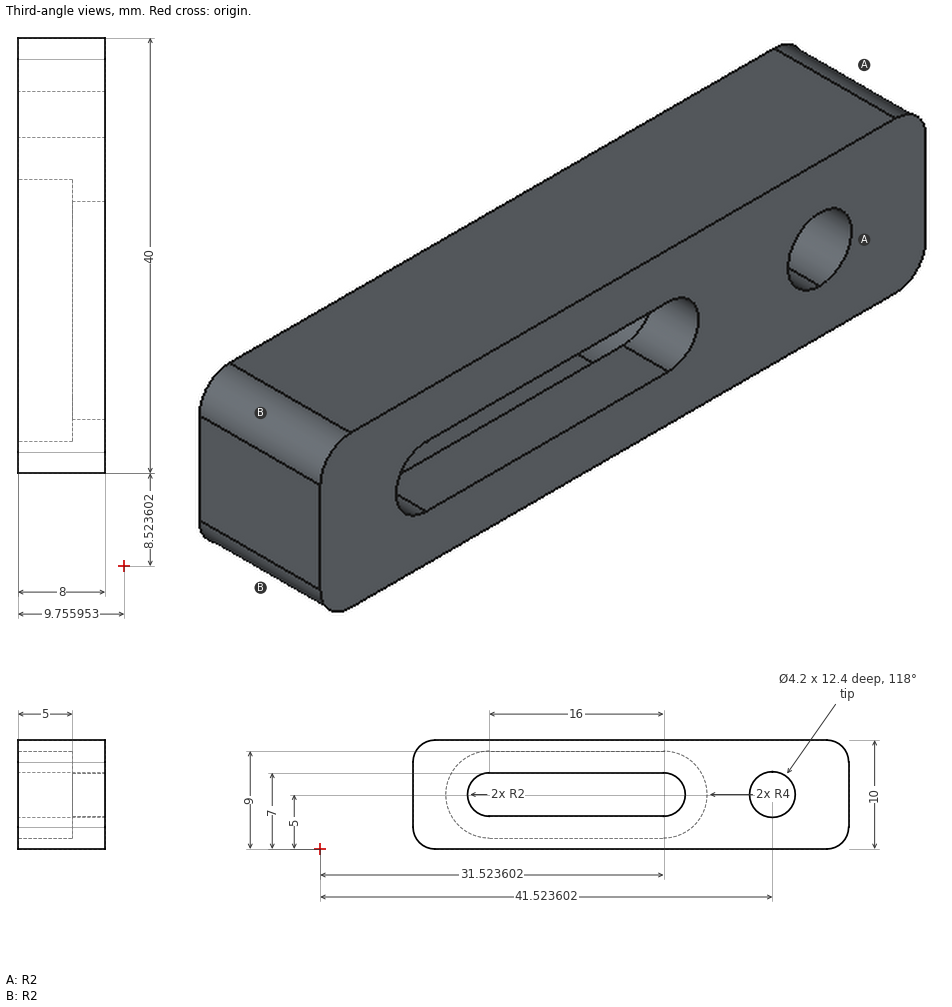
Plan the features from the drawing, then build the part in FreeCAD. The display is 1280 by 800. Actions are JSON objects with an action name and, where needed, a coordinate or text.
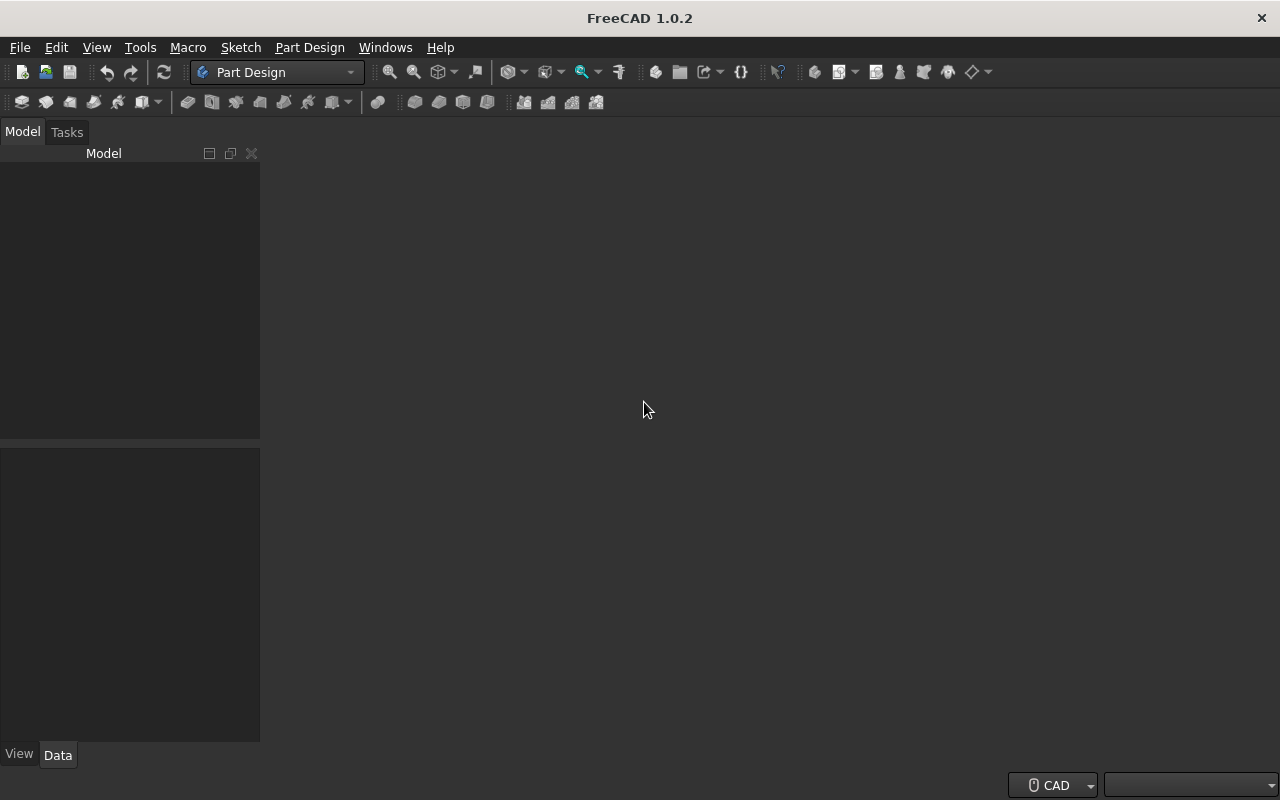
{"action": "left_click", "coordinate": [22, 72]}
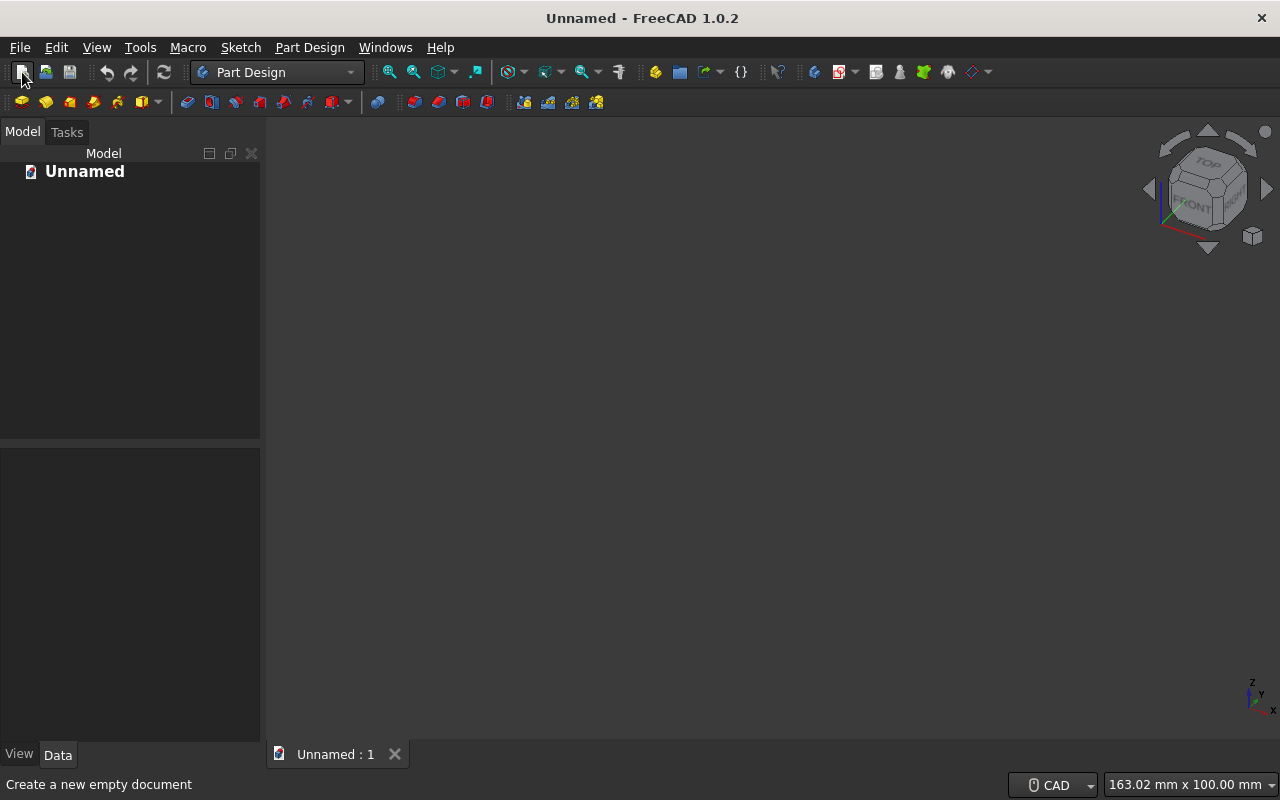
{"action": "left_click", "coordinate": [840, 72]}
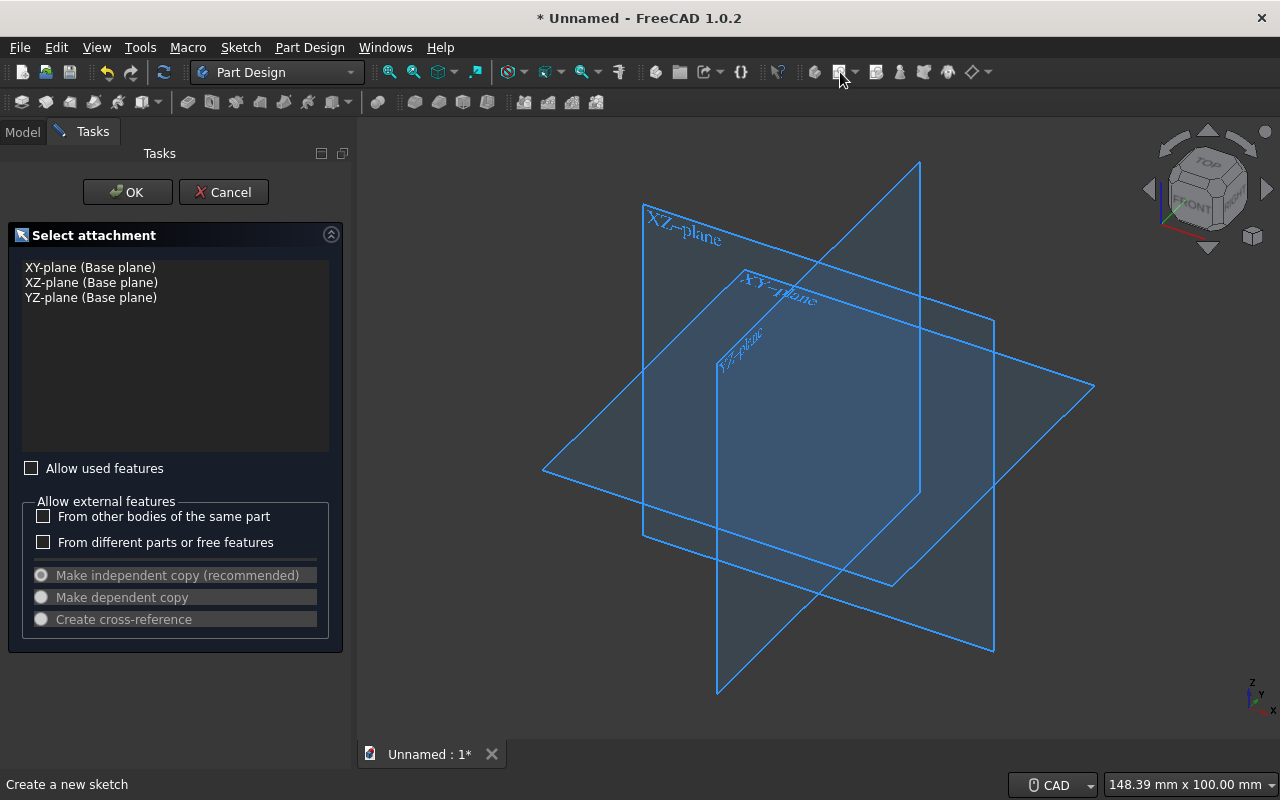
{"action": "left_click", "coordinate": [82, 268]}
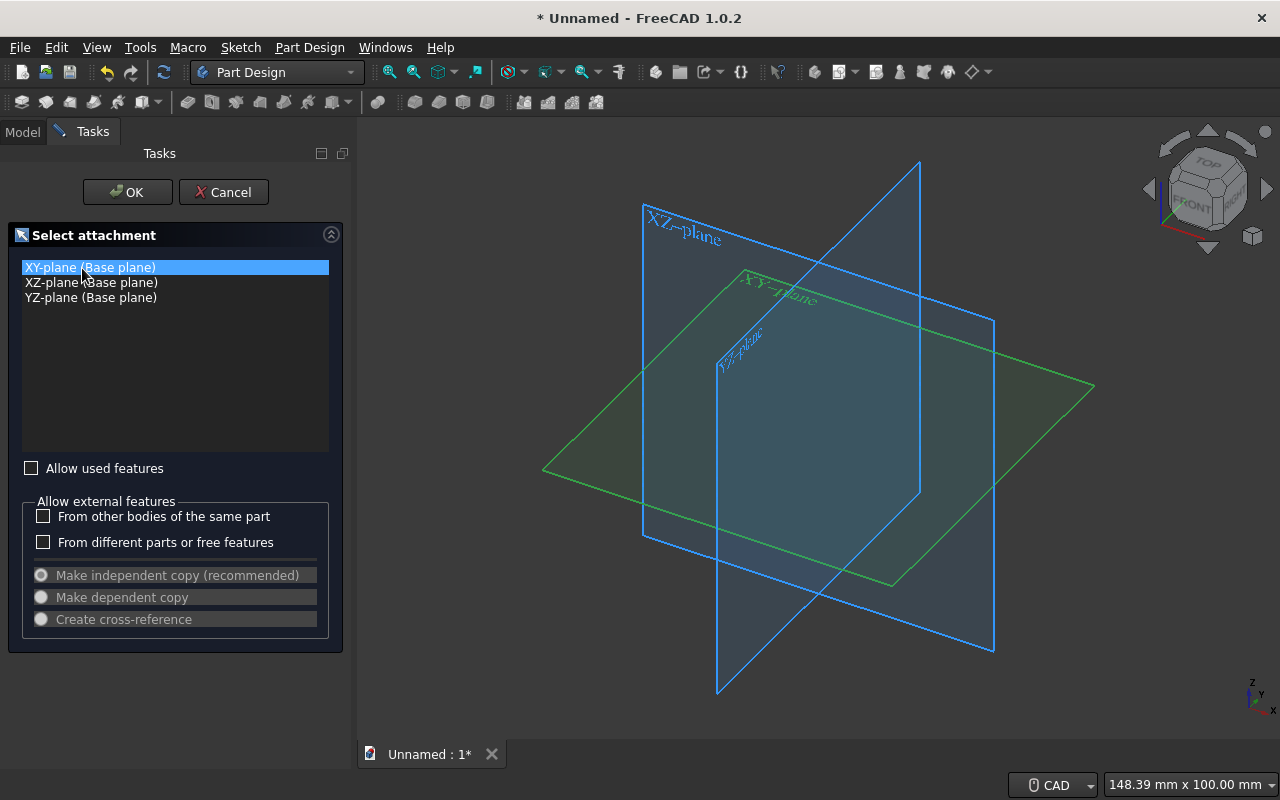
{"action": "left_click", "coordinate": [128, 192]}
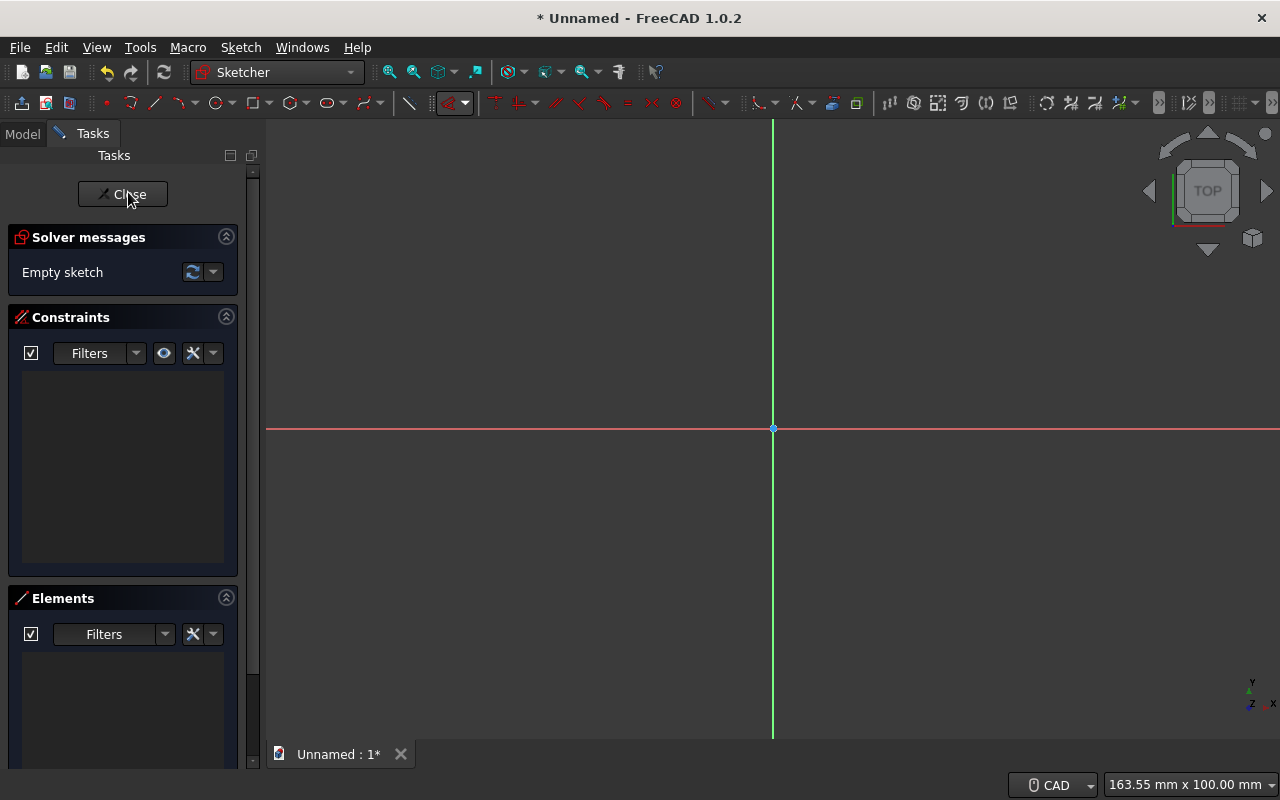
{"action": "scroll", "coordinate": [532, 711], "scroll_direction": "down", "scroll_amount": 1}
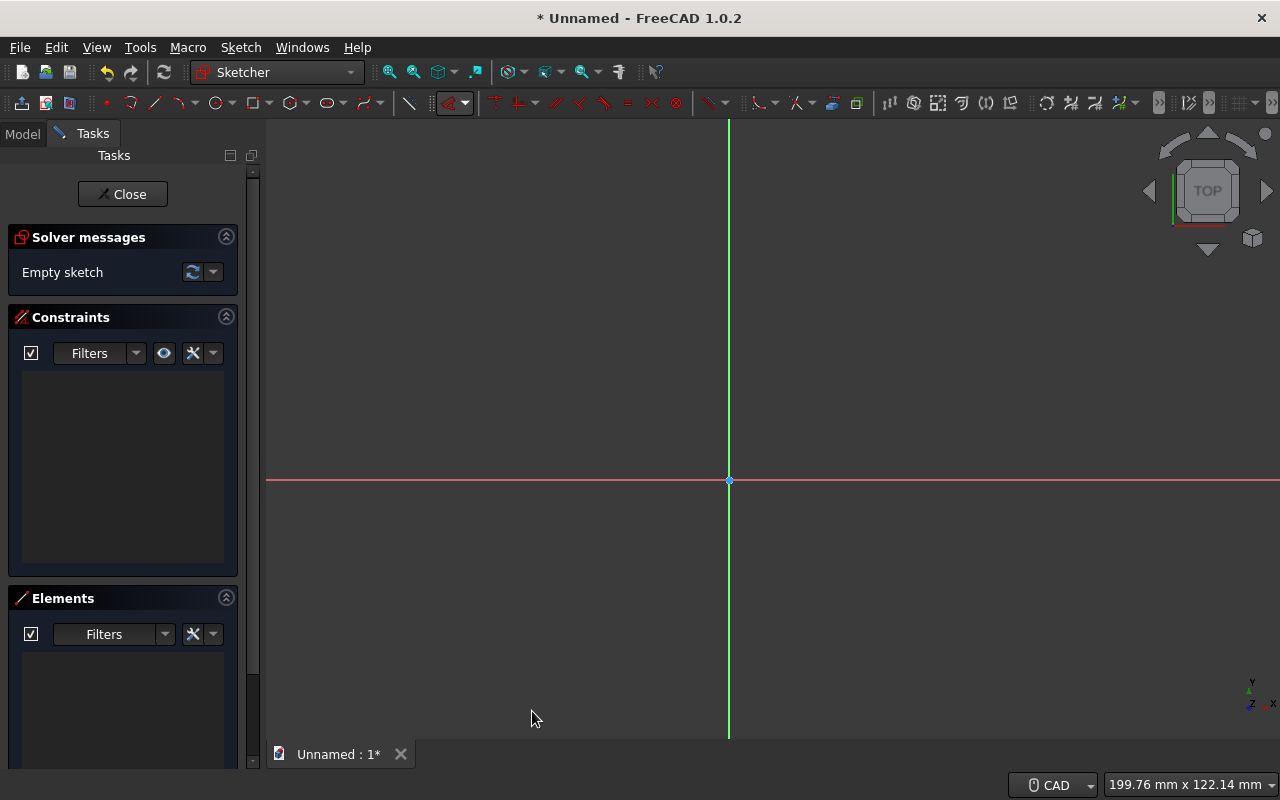
{"action": "scroll", "coordinate": [705, 211], "scroll_direction": "up", "scroll_amount": 2}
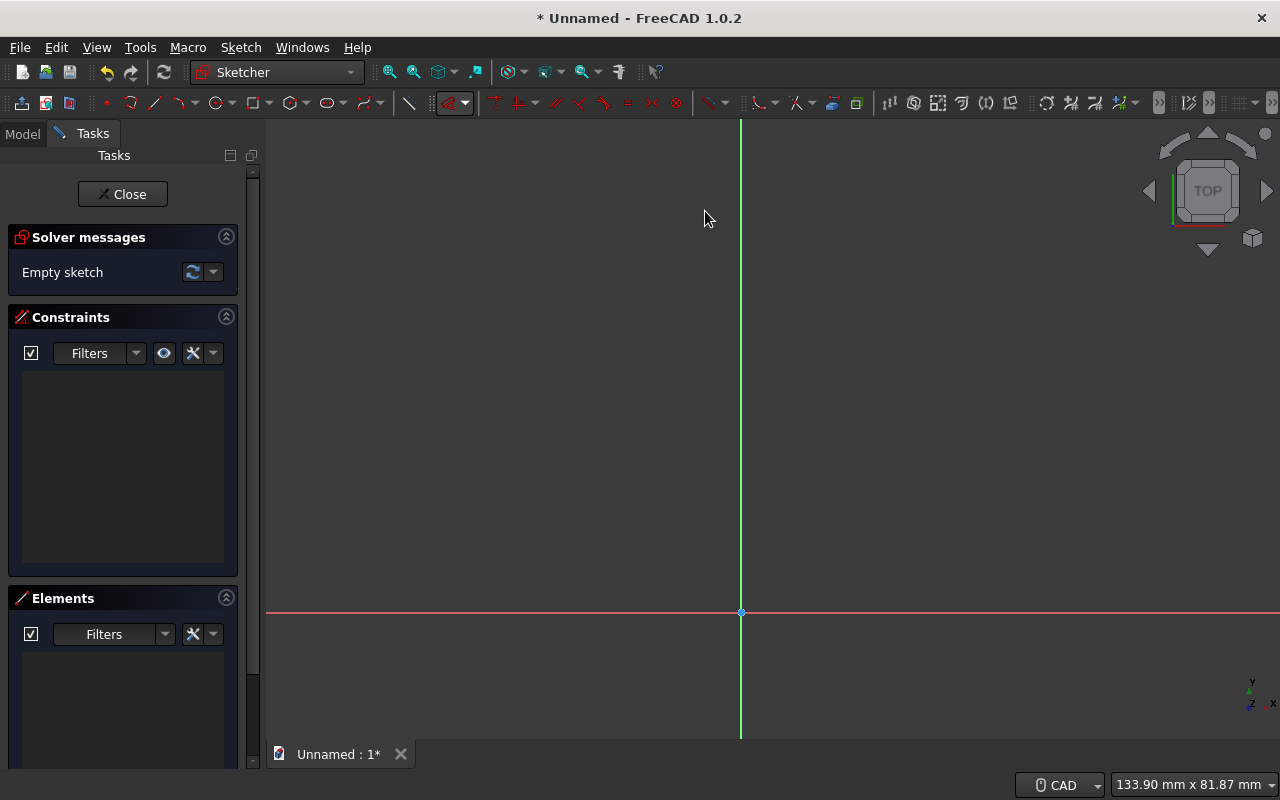
{"action": "key", "text": "g r"}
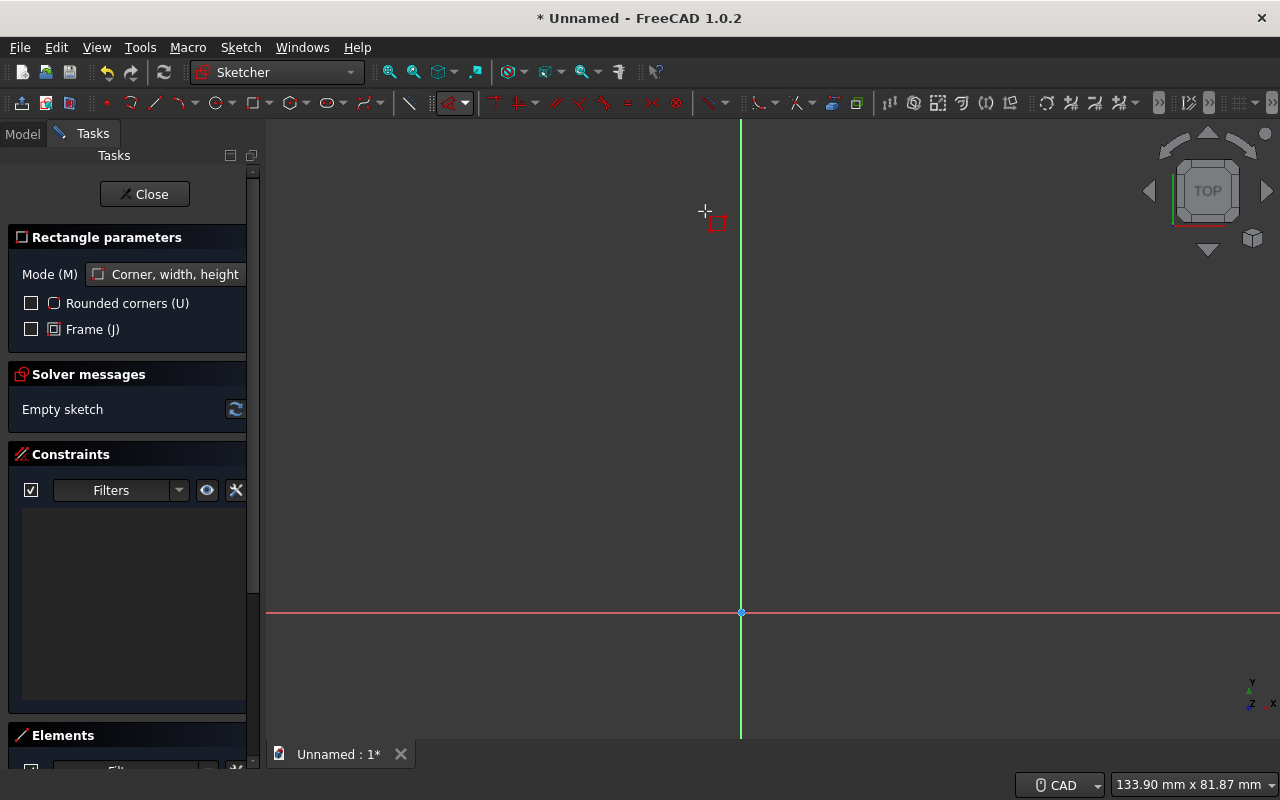
{"action": "left_click", "coordinate": [667, 245]}
{"action": "mouse_move", "coordinate": [728, 548]}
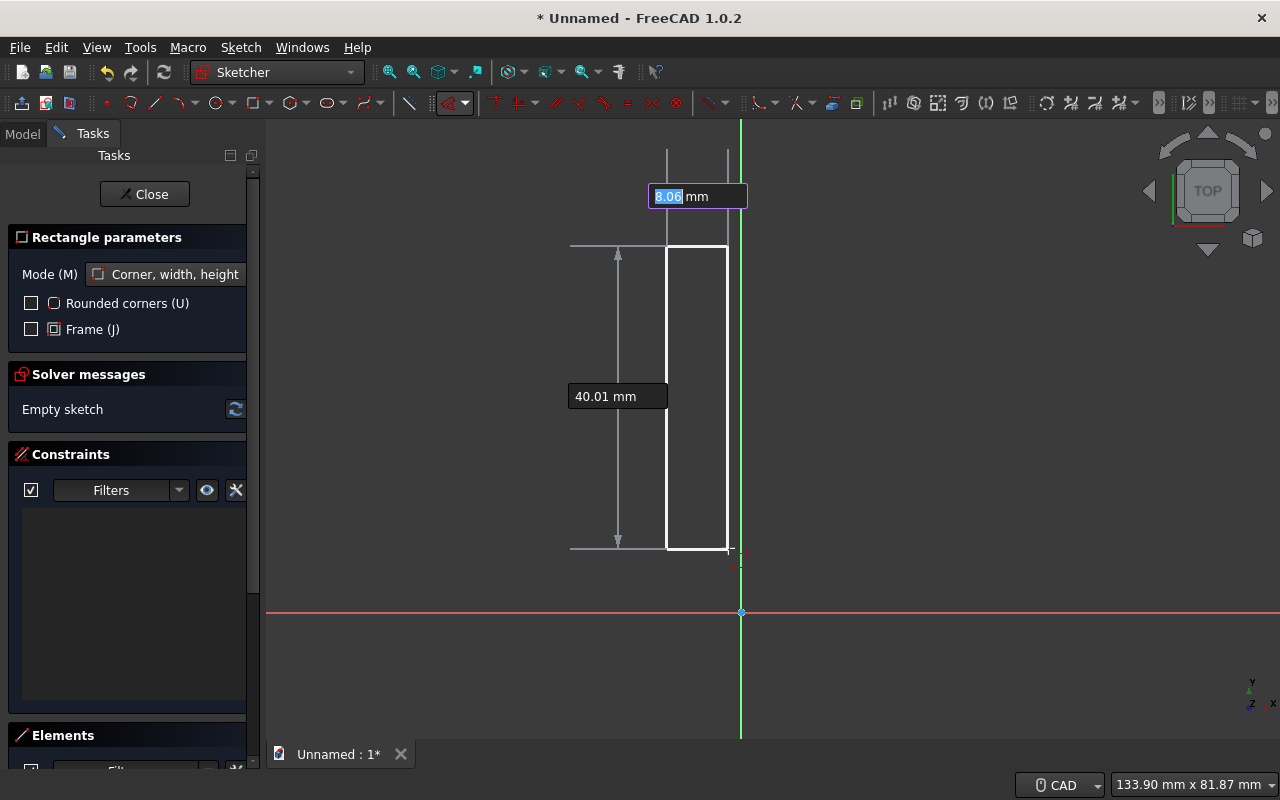
{"action": "type", "text": "8"}
{"action": "key", "text": "Tab"}
{"action": "type", "text": "40"}
{"action": "key", "text": "Return"}
{"action": "key", "text": "Escape"}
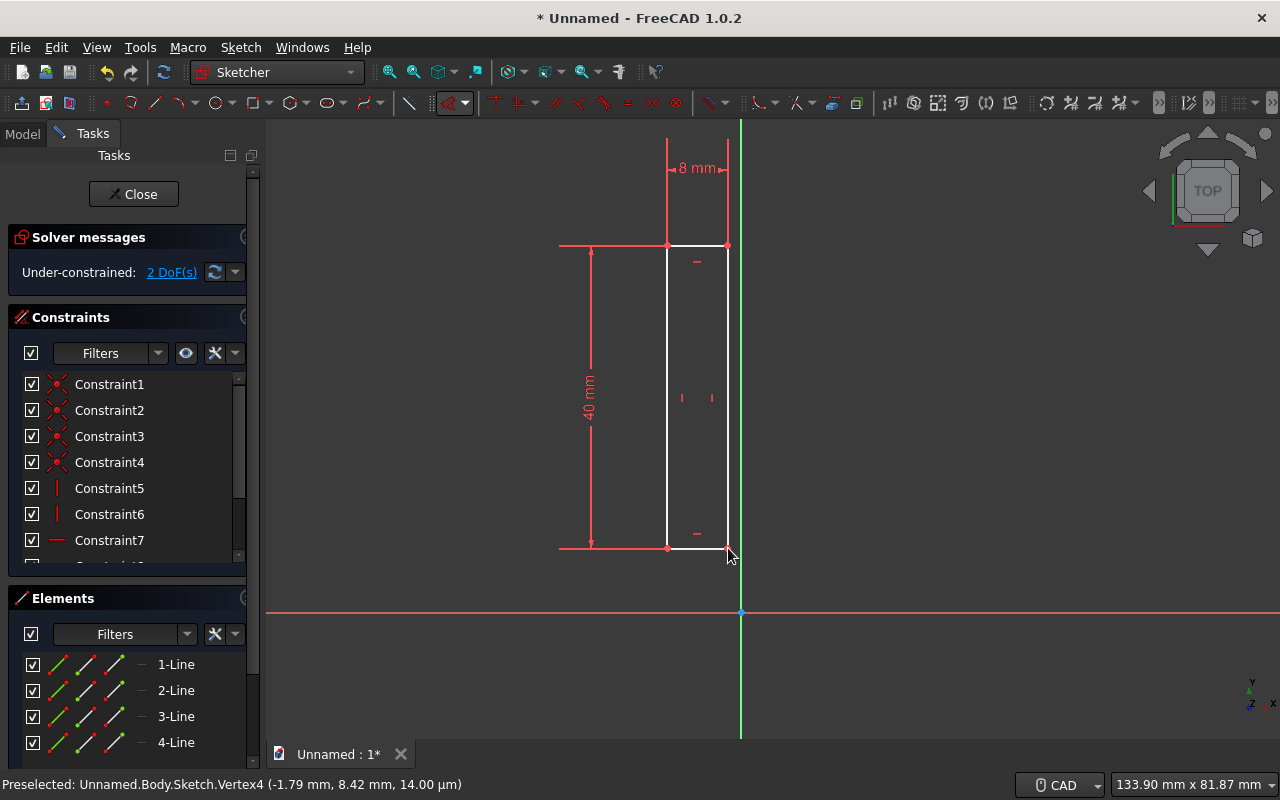
{"action": "key", "text": "d"}